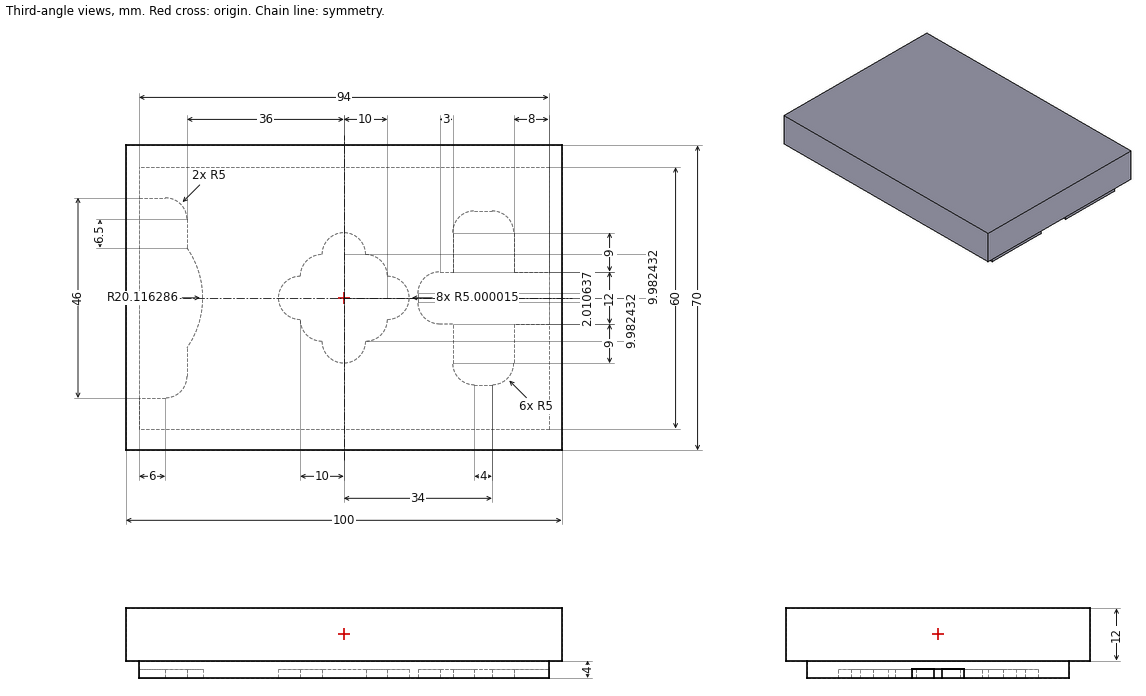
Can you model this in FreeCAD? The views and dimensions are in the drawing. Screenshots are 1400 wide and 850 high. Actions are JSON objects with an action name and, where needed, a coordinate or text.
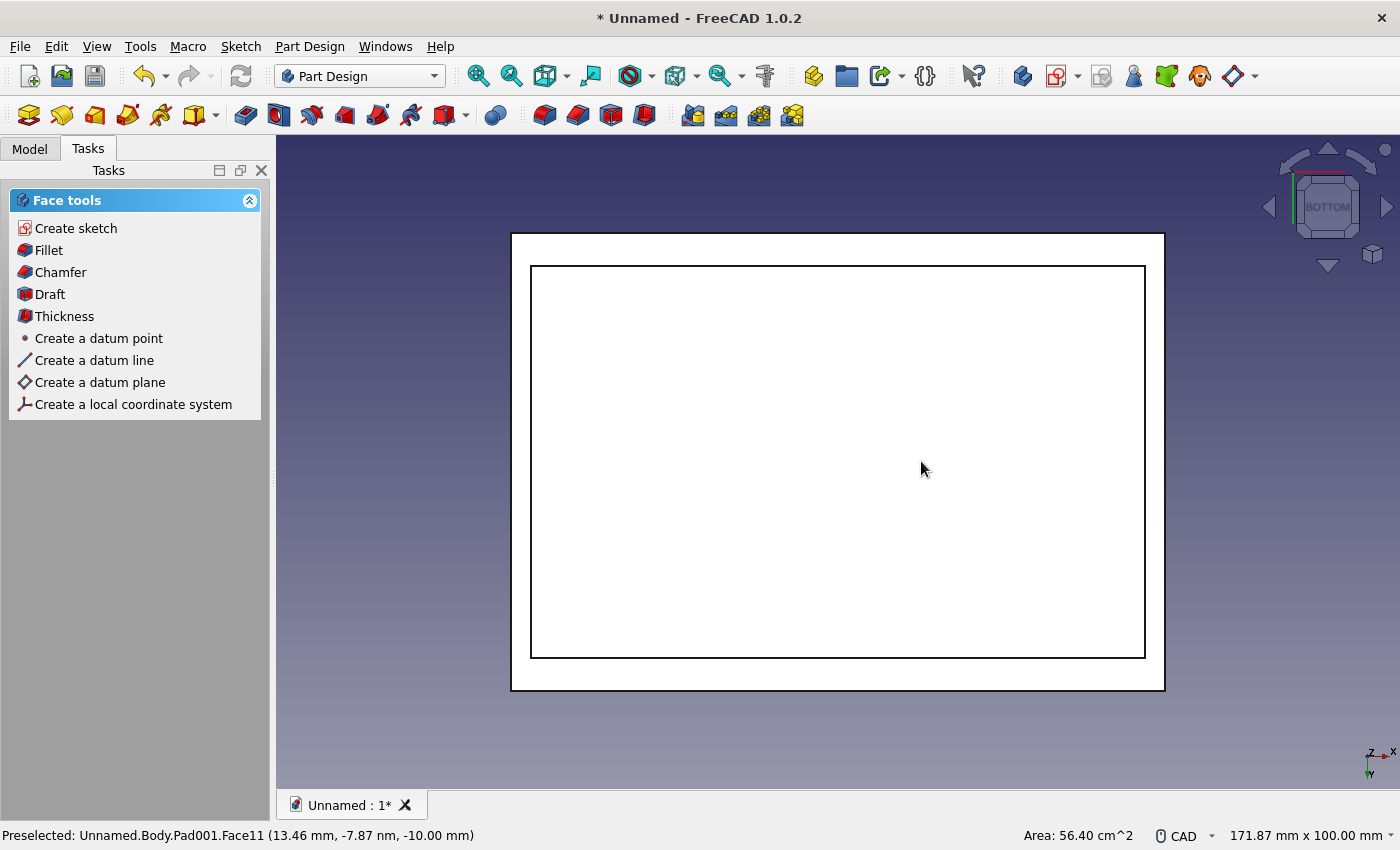
{"action": "left_click", "coordinate": [1056, 76]}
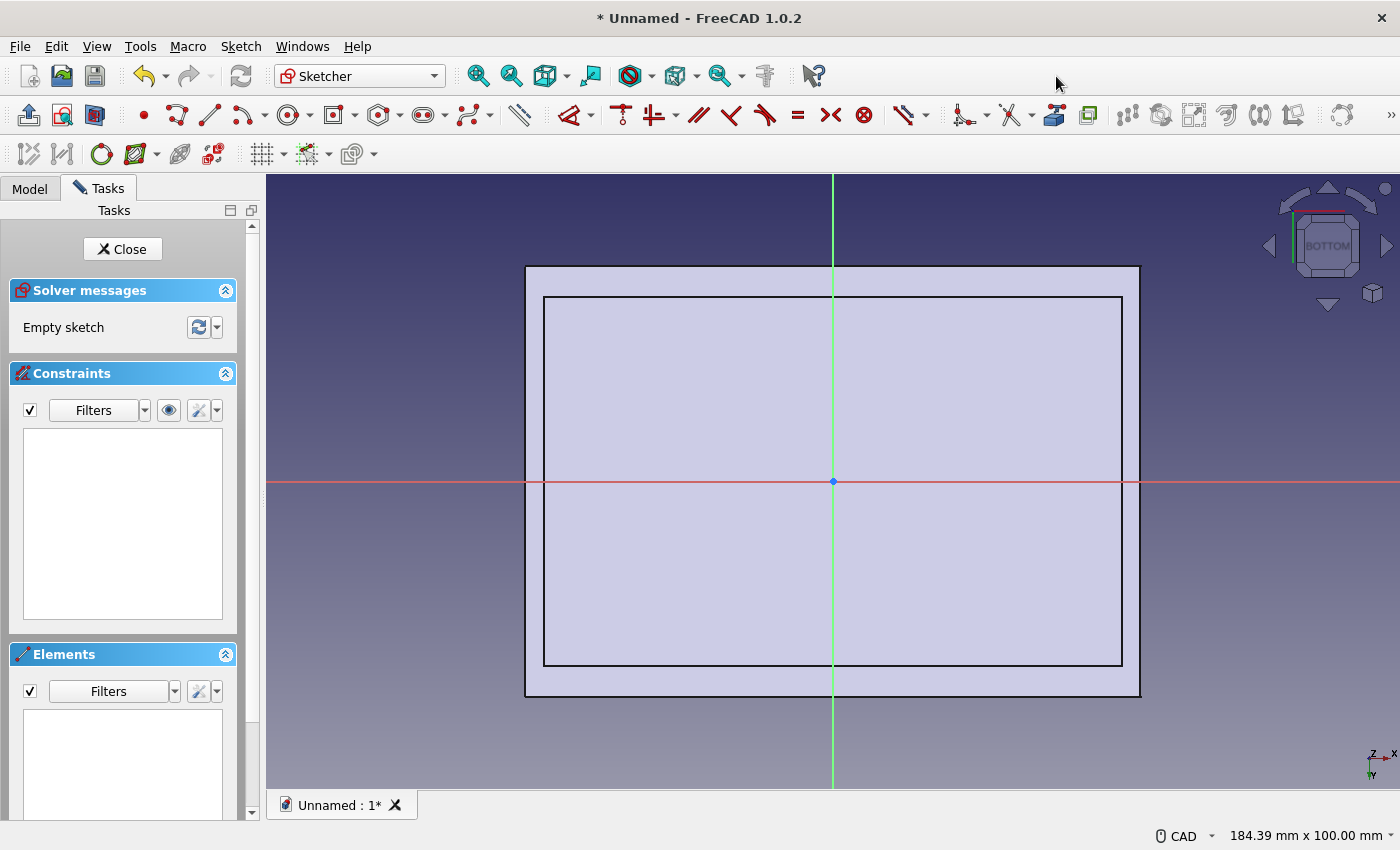
{"action": "scroll", "coordinate": [534, 482], "scroll_direction": "up", "scroll_amount": 2}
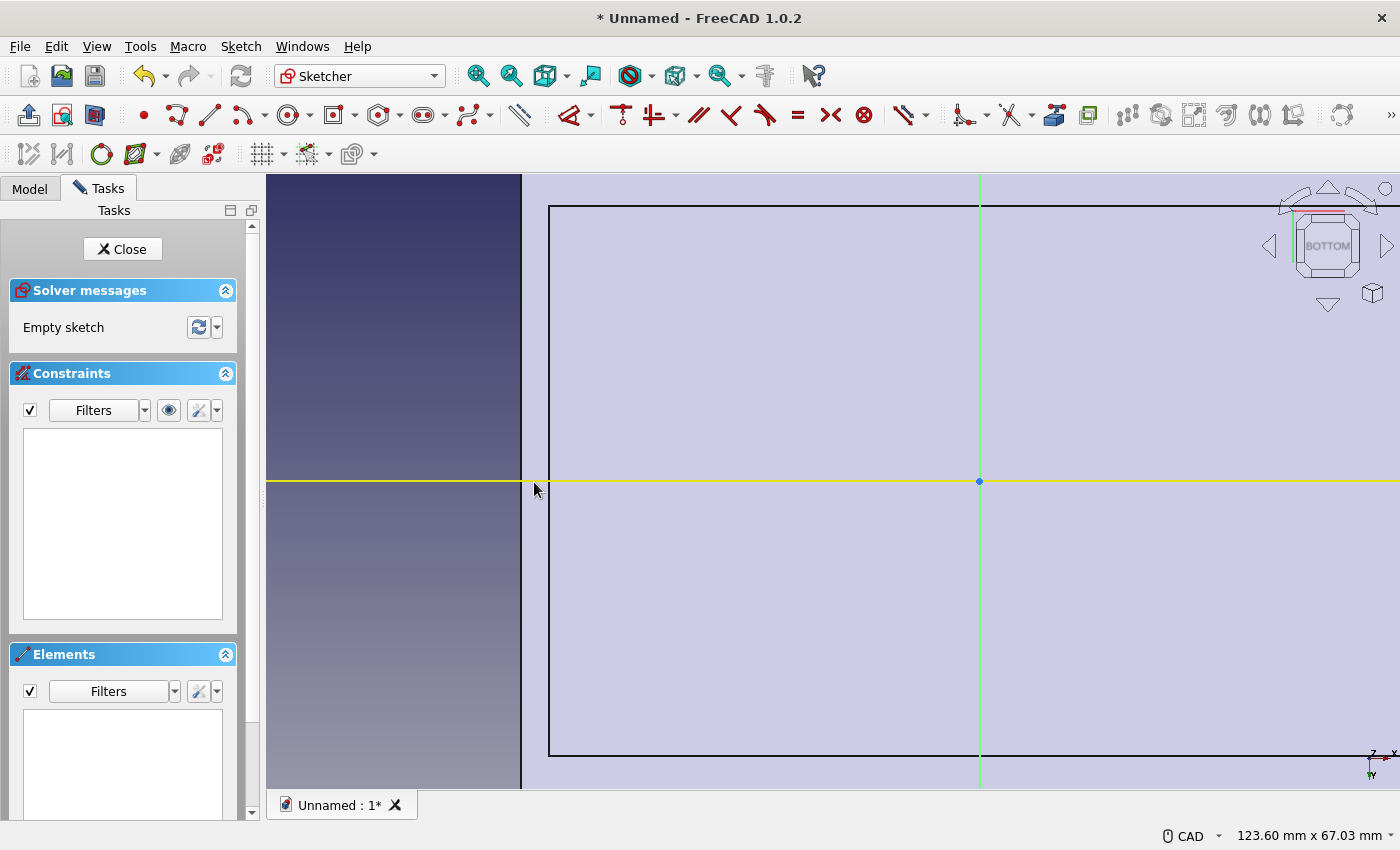
{"action": "left_click", "coordinate": [210, 116]}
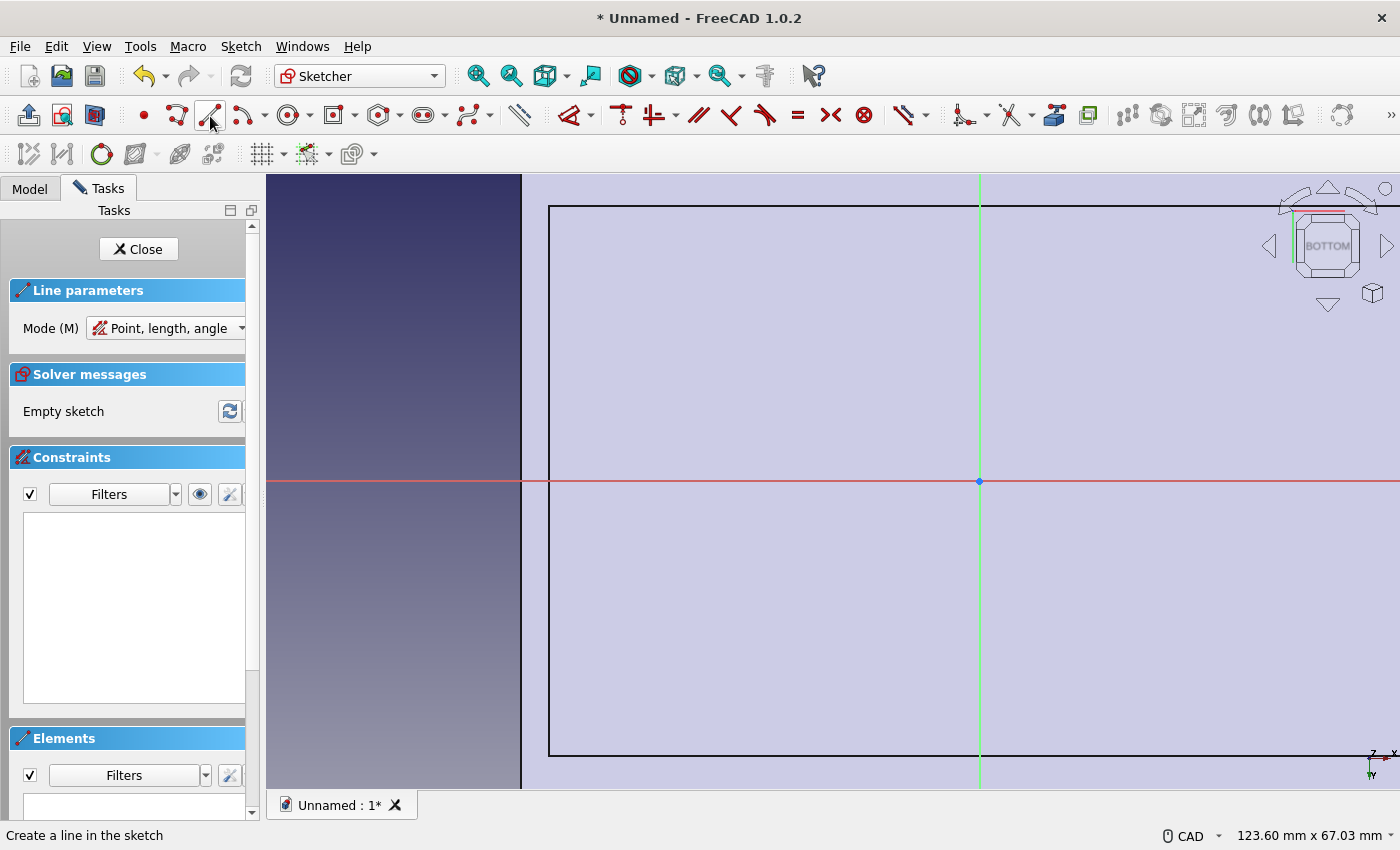
{"action": "left_click", "coordinate": [650, 646]}
{"action": "left_click", "coordinate": [650, 587]}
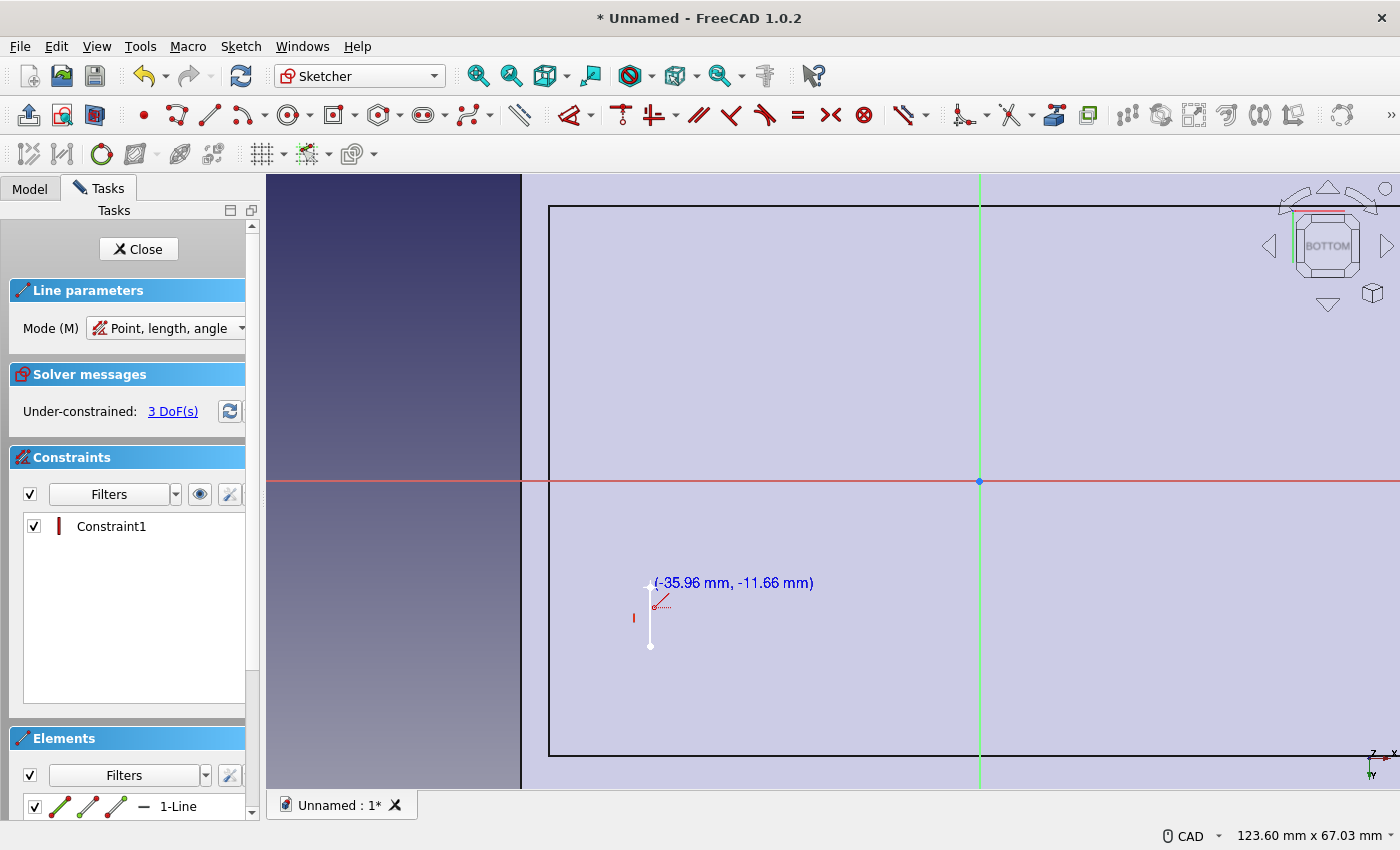
{"action": "left_click", "coordinate": [650, 375]}
{"action": "left_click", "coordinate": [650, 316]}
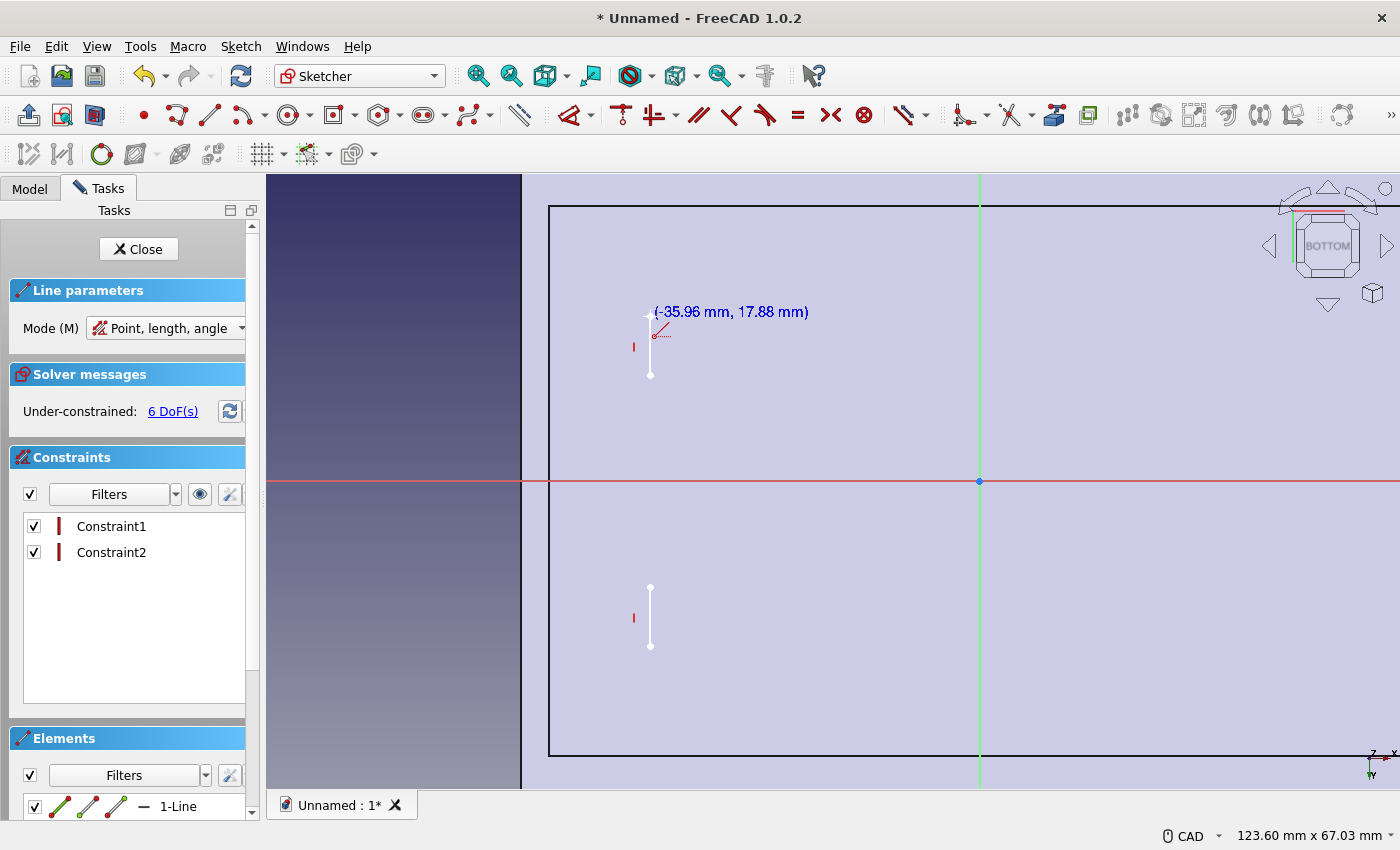
{"action": "left_click", "coordinate": [177, 116]}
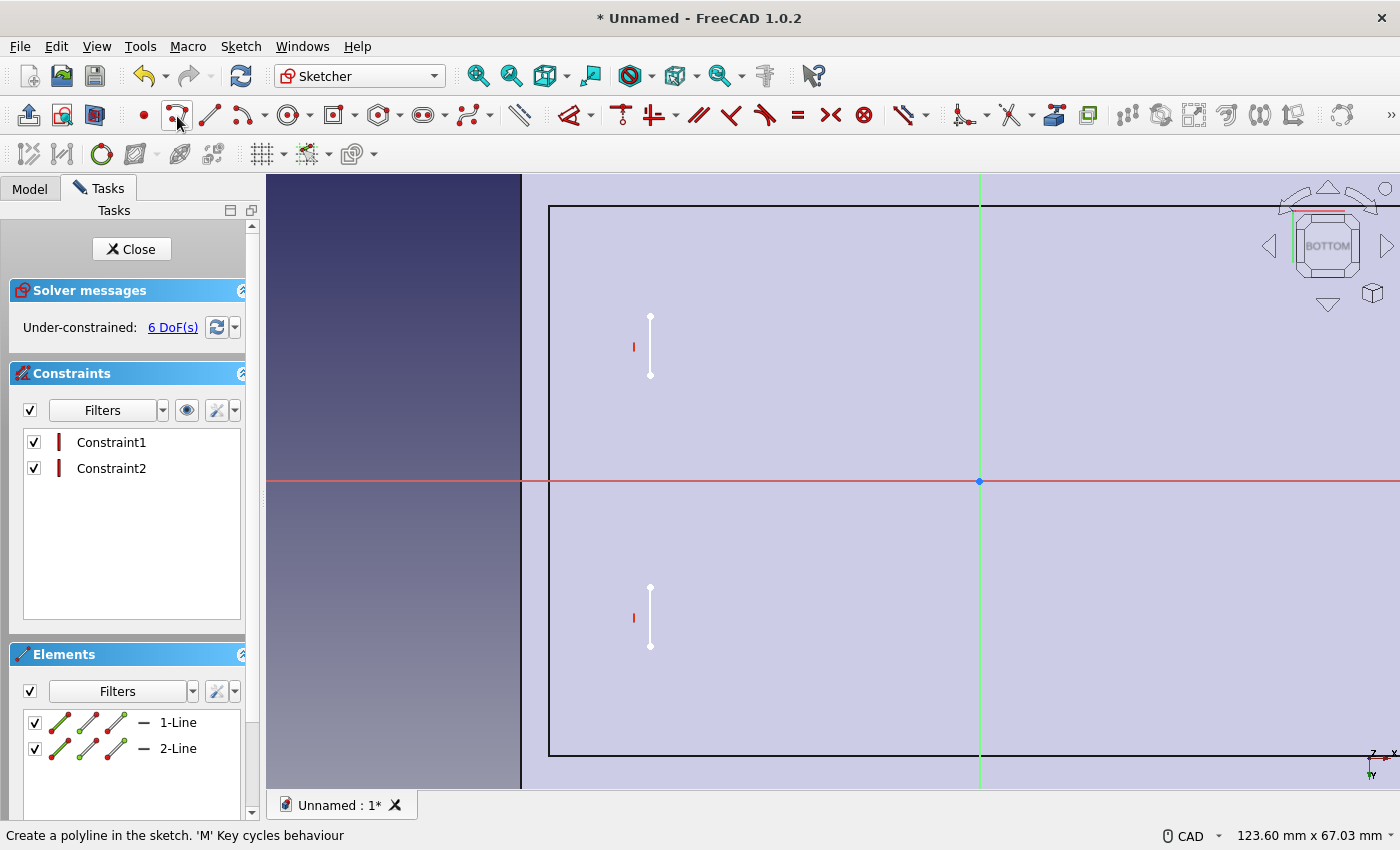
{"action": "left_click", "coordinate": [604, 270]}
{"action": "left_click", "coordinate": [549, 270]}
{"action": "left_click", "coordinate": [549, 692]}
{"action": "left_click", "coordinate": [604, 692]}
{"action": "right_click", "coordinate": [604, 692]}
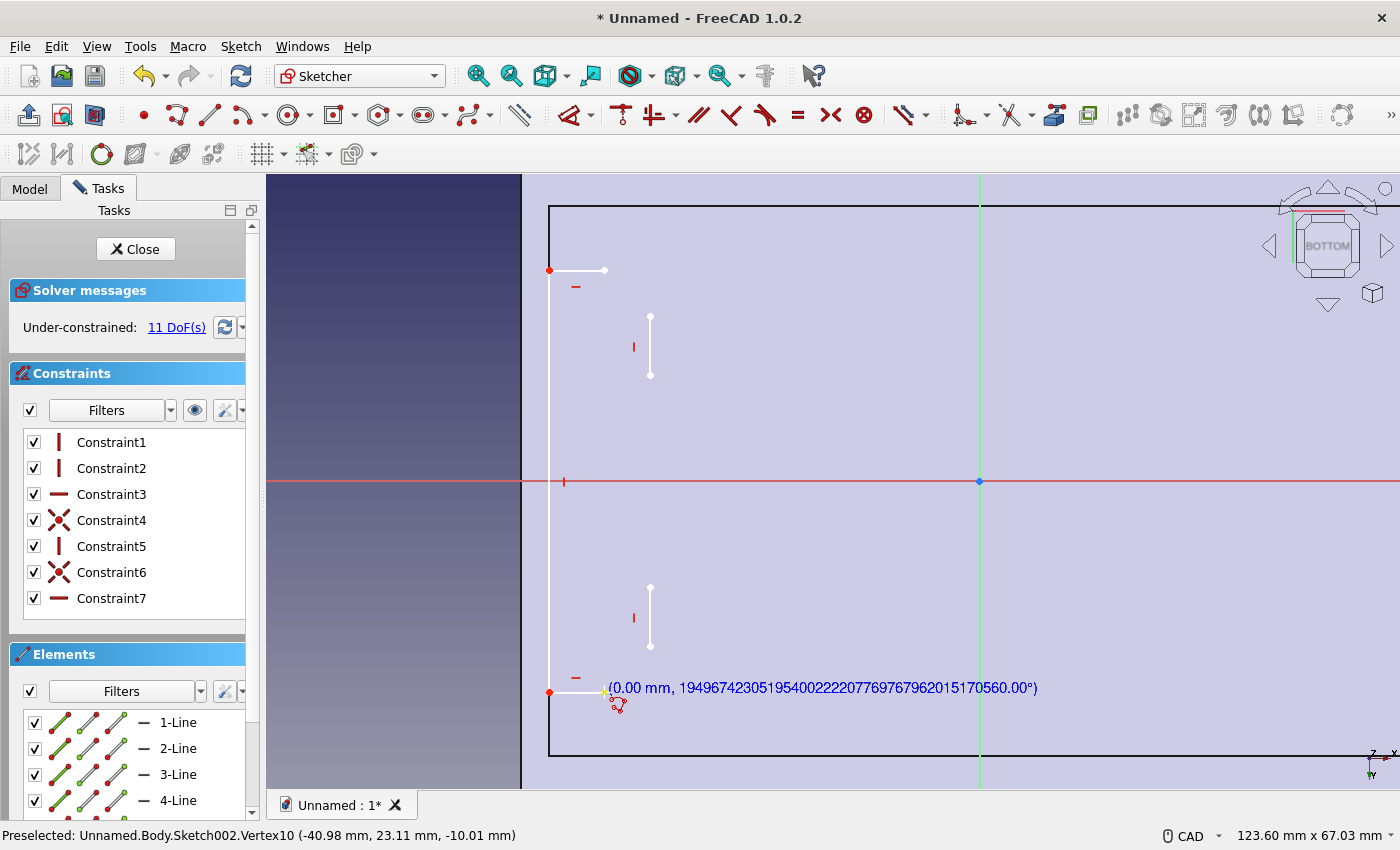
{"action": "key", "text": "g 3 a"}